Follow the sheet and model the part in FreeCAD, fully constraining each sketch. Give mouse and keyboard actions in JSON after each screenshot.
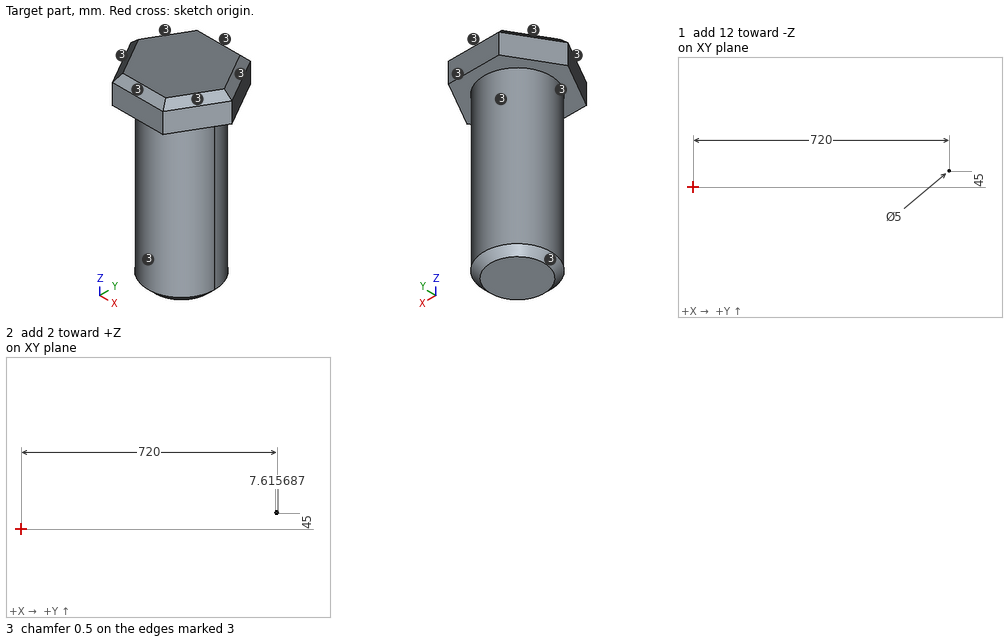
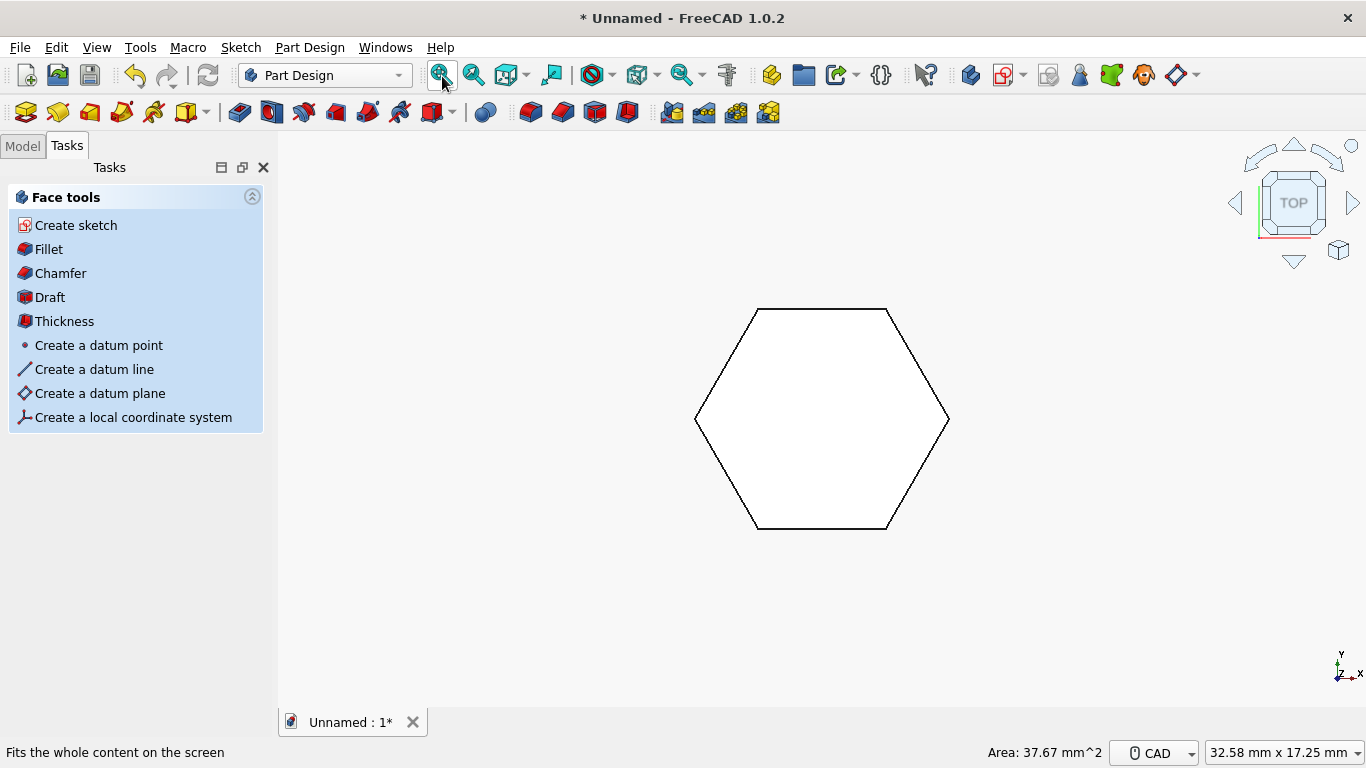
{"action": "key", "text": "1"}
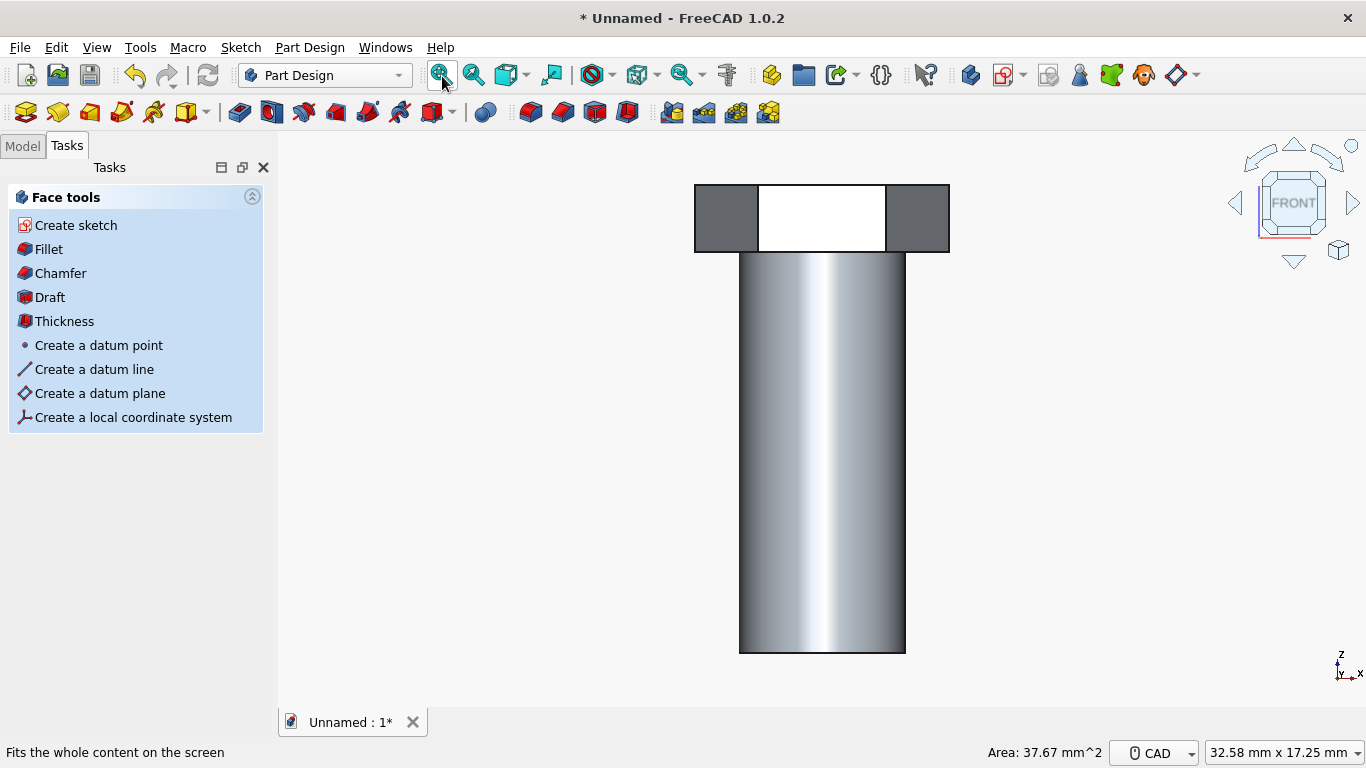
{"action": "left_click", "coordinate": [739, 652], "text": "ctrl"}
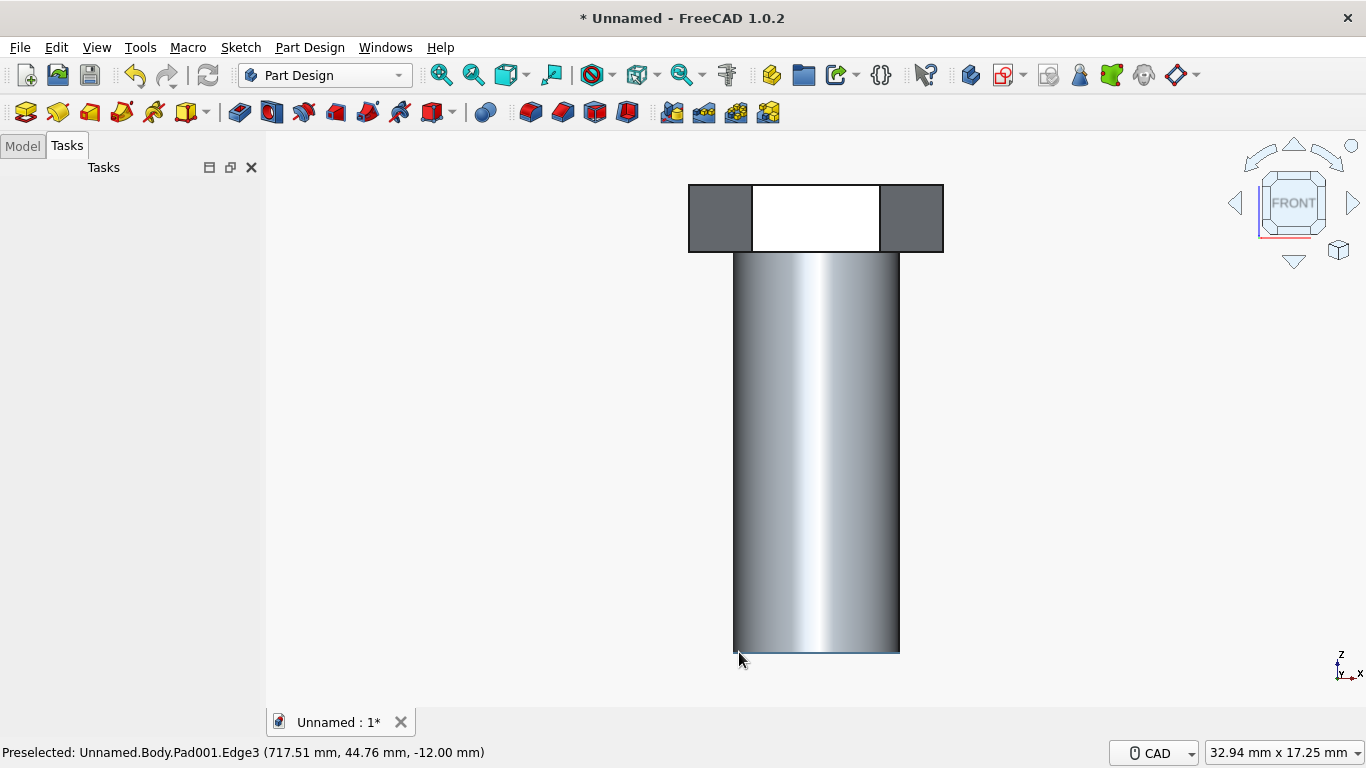
{"action": "left_click", "coordinate": [564, 112]}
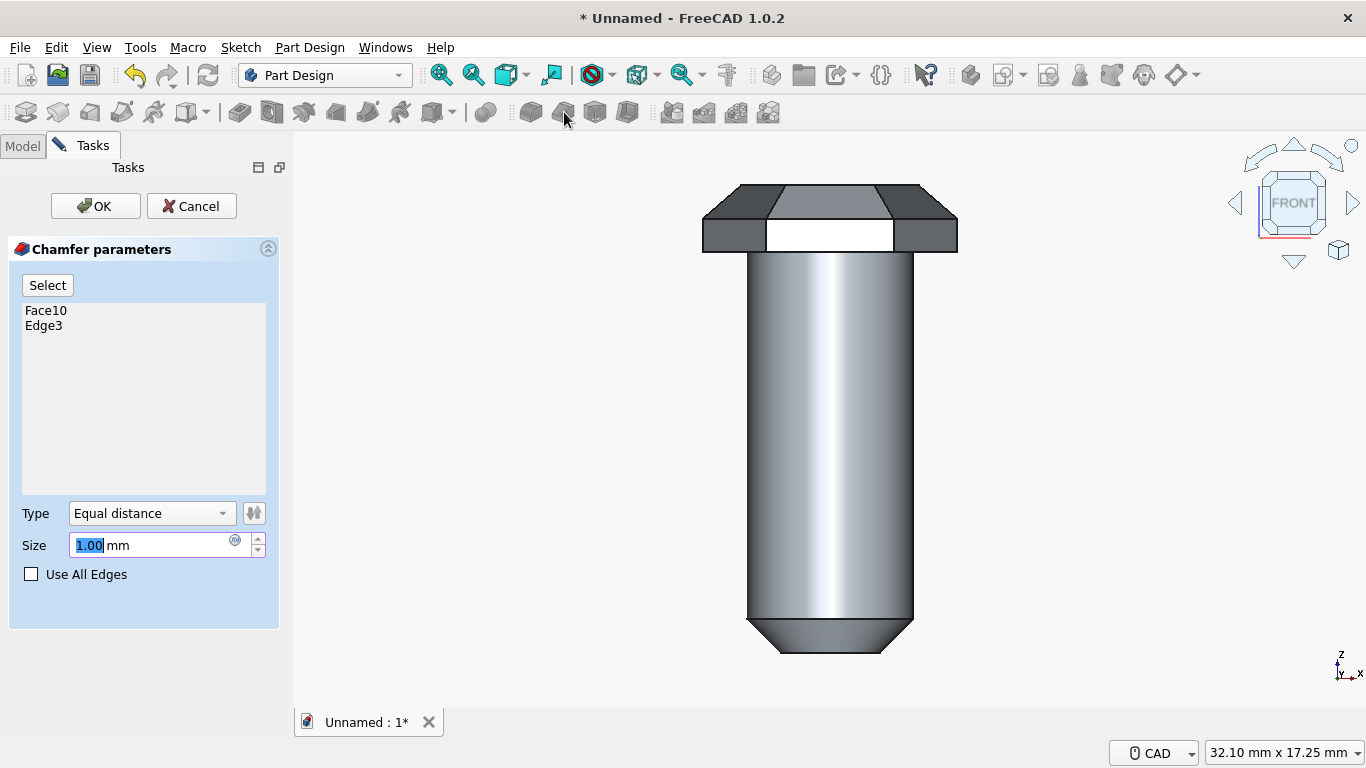
{"action": "type", "text": "0.5"}
{"action": "key", "text": "Tab"}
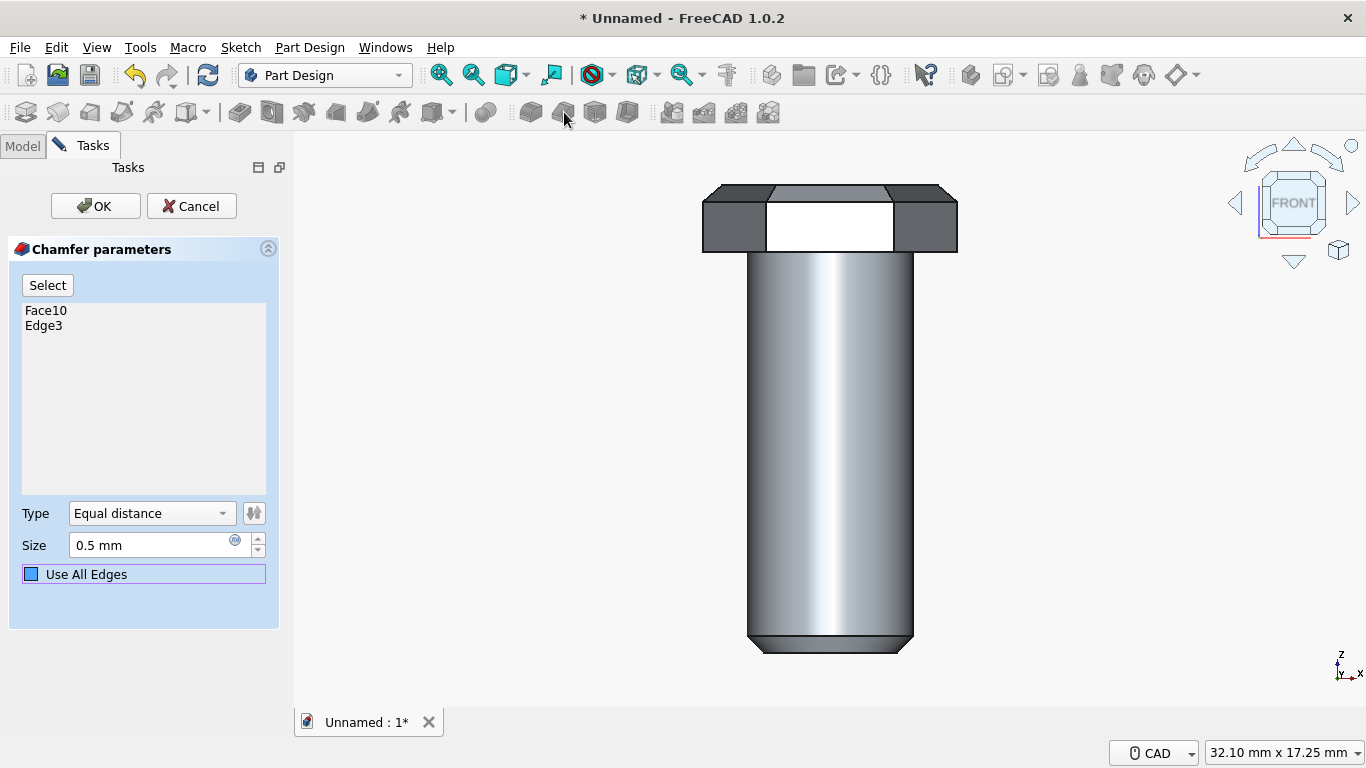
{"action": "left_click", "coordinate": [96, 206]}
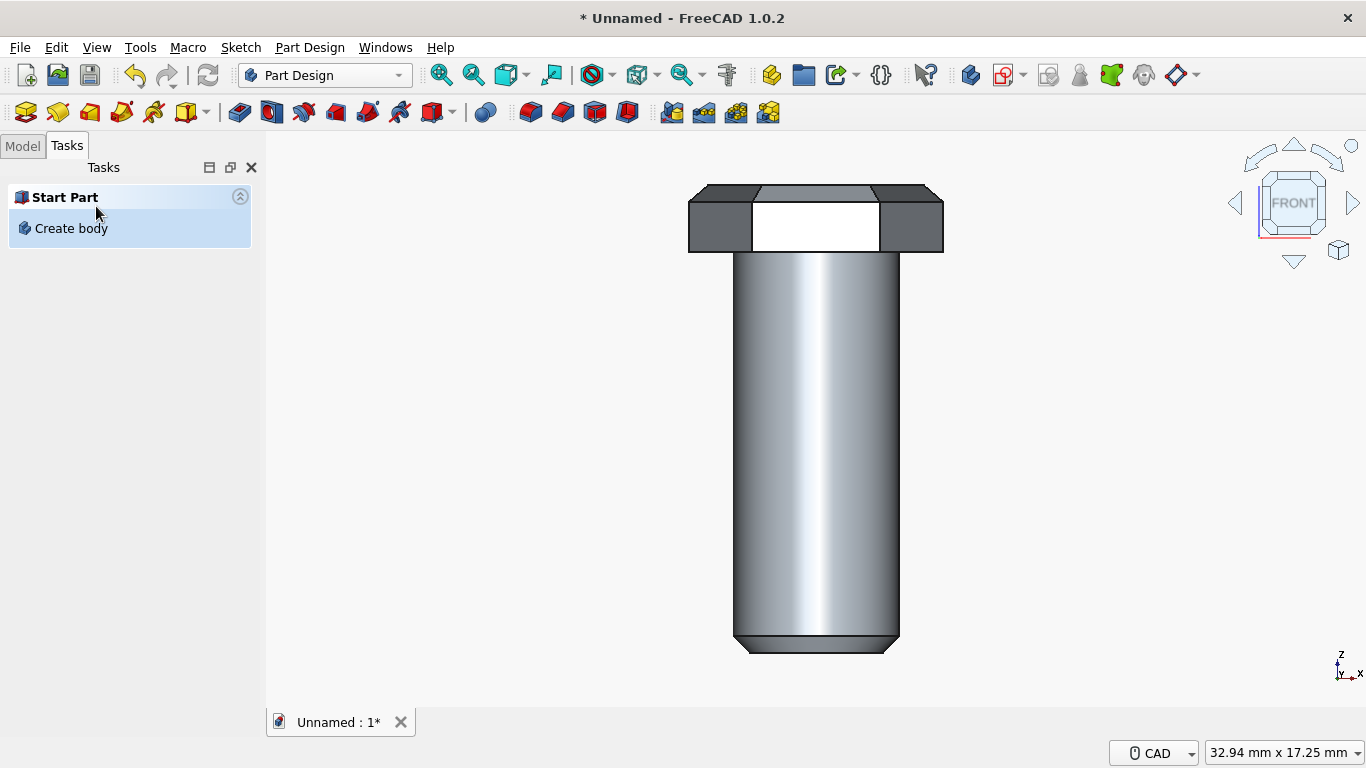
{"action": "key", "text": "0"}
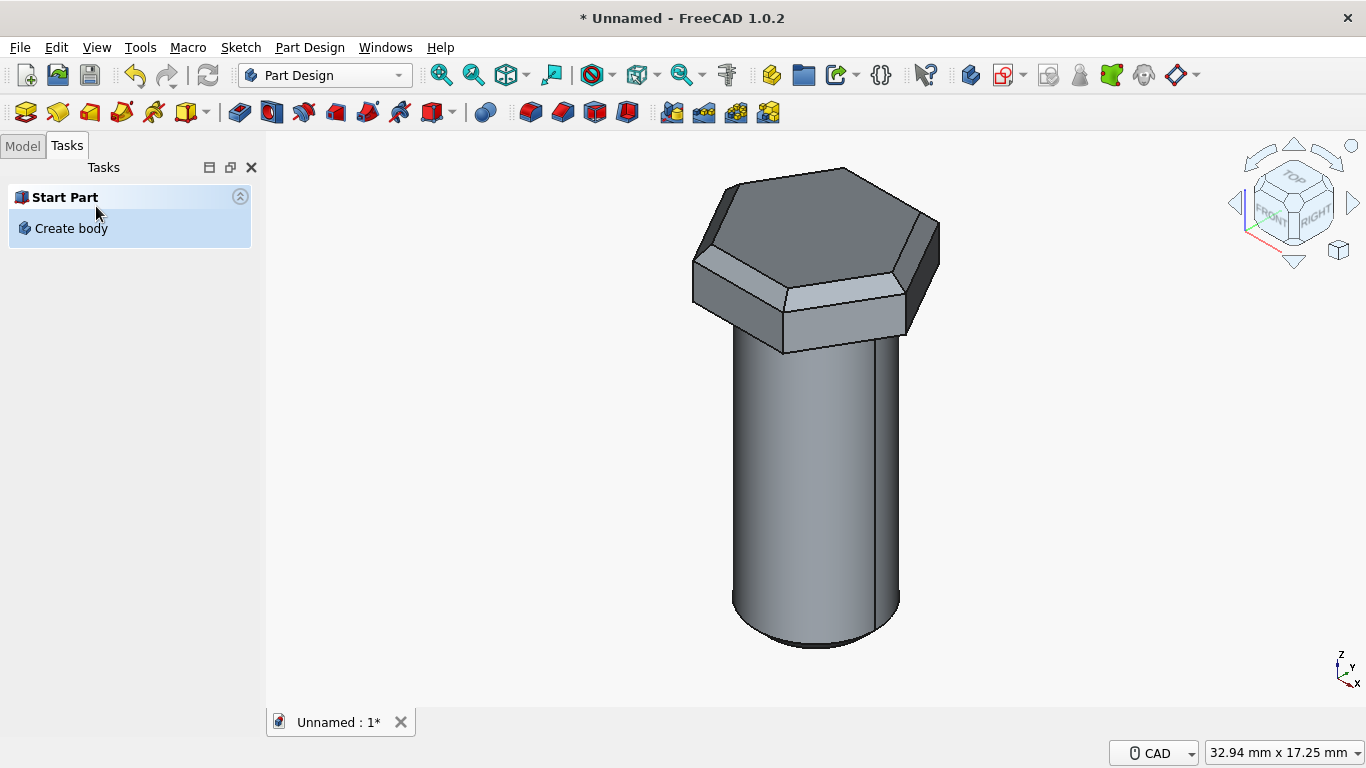
{"action": "left_click", "coordinate": [442, 76]}